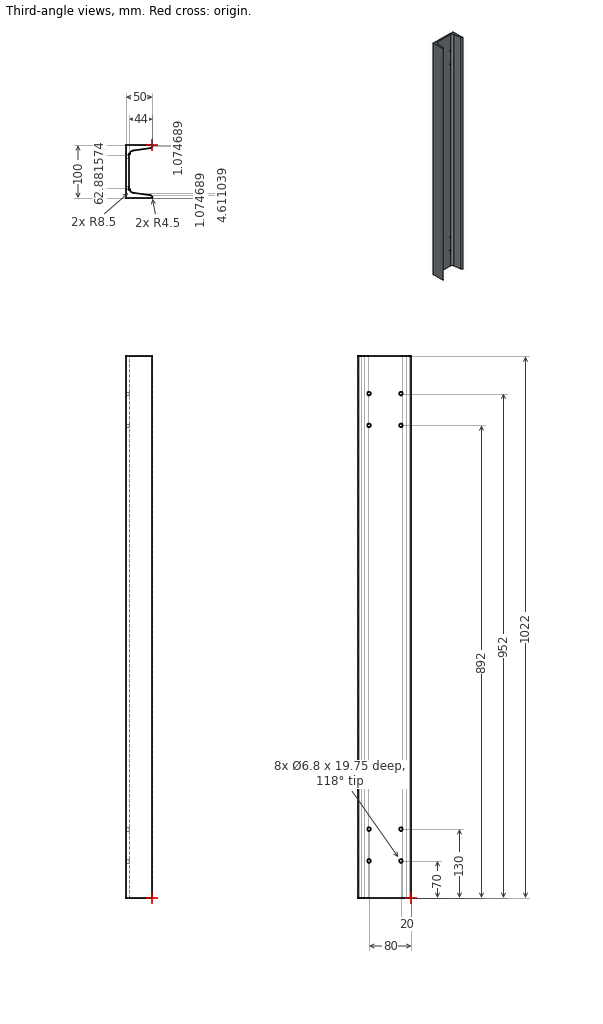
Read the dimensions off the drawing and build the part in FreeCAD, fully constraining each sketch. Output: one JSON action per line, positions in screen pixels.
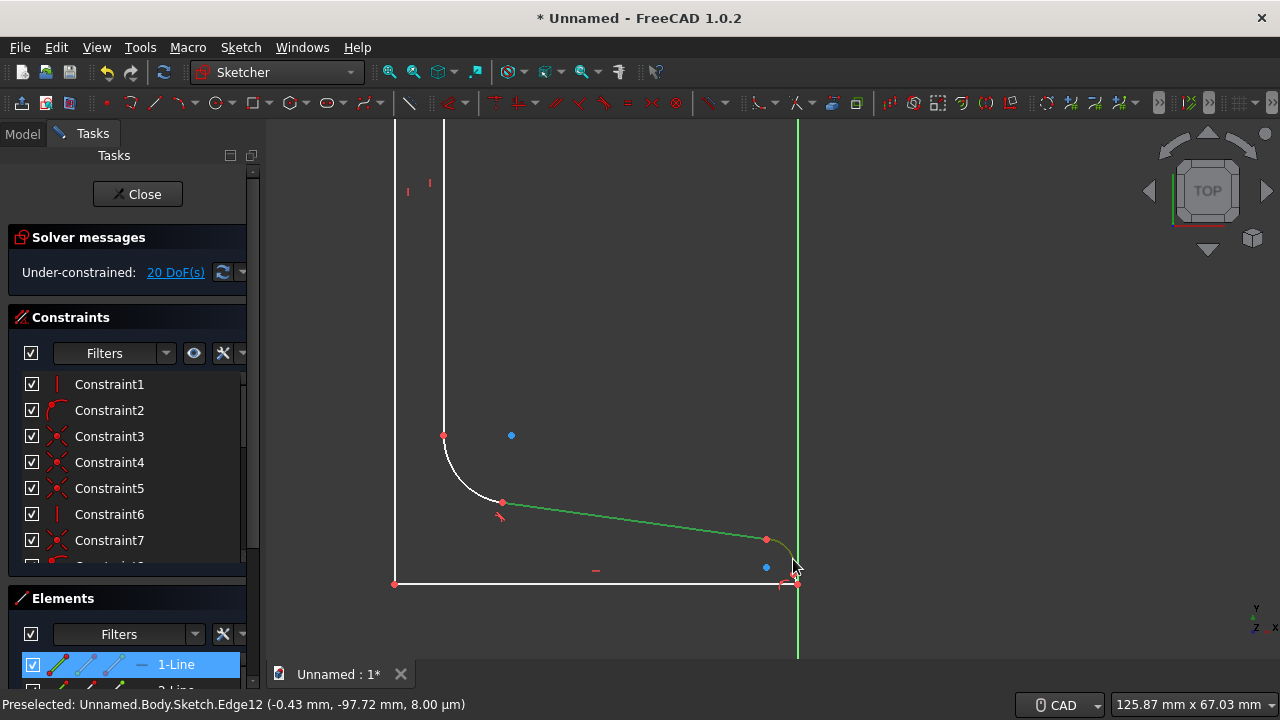
{"action": "key", "text": "t"}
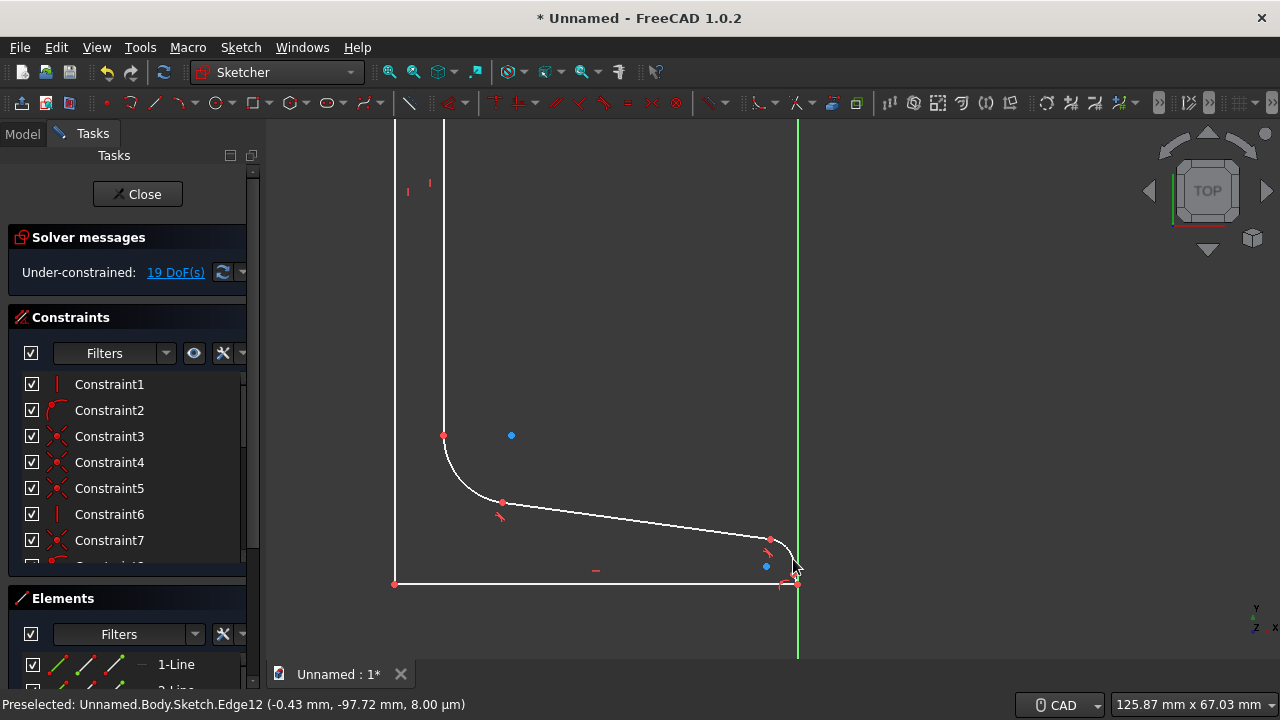
{"action": "left_click", "coordinate": [444, 283]}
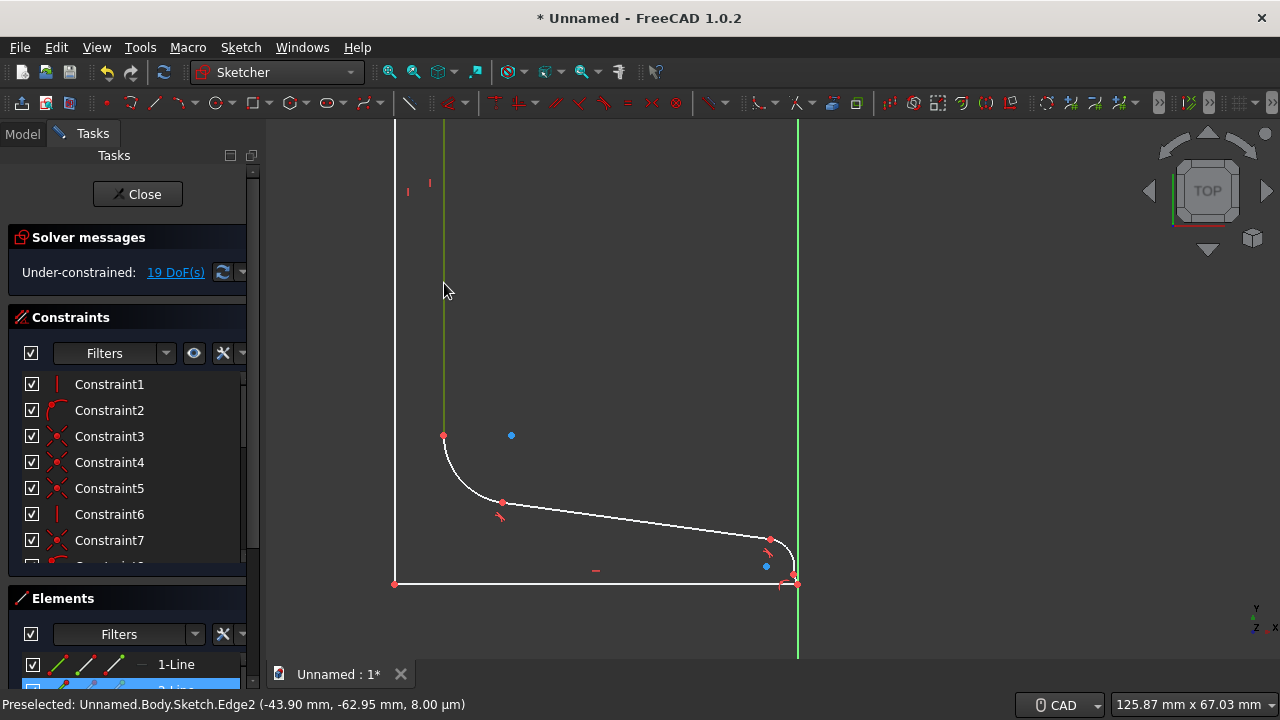
{"action": "left_click", "coordinate": [450, 464]}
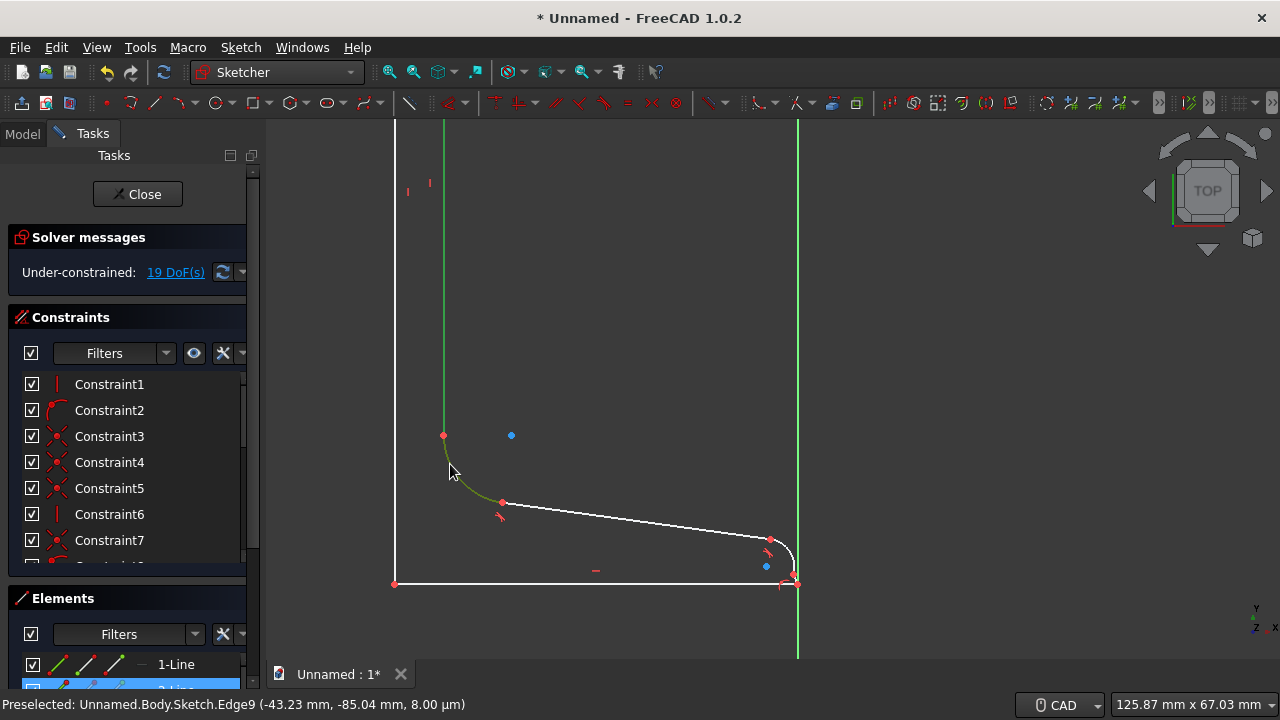
{"action": "left_click", "coordinate": [604, 104]}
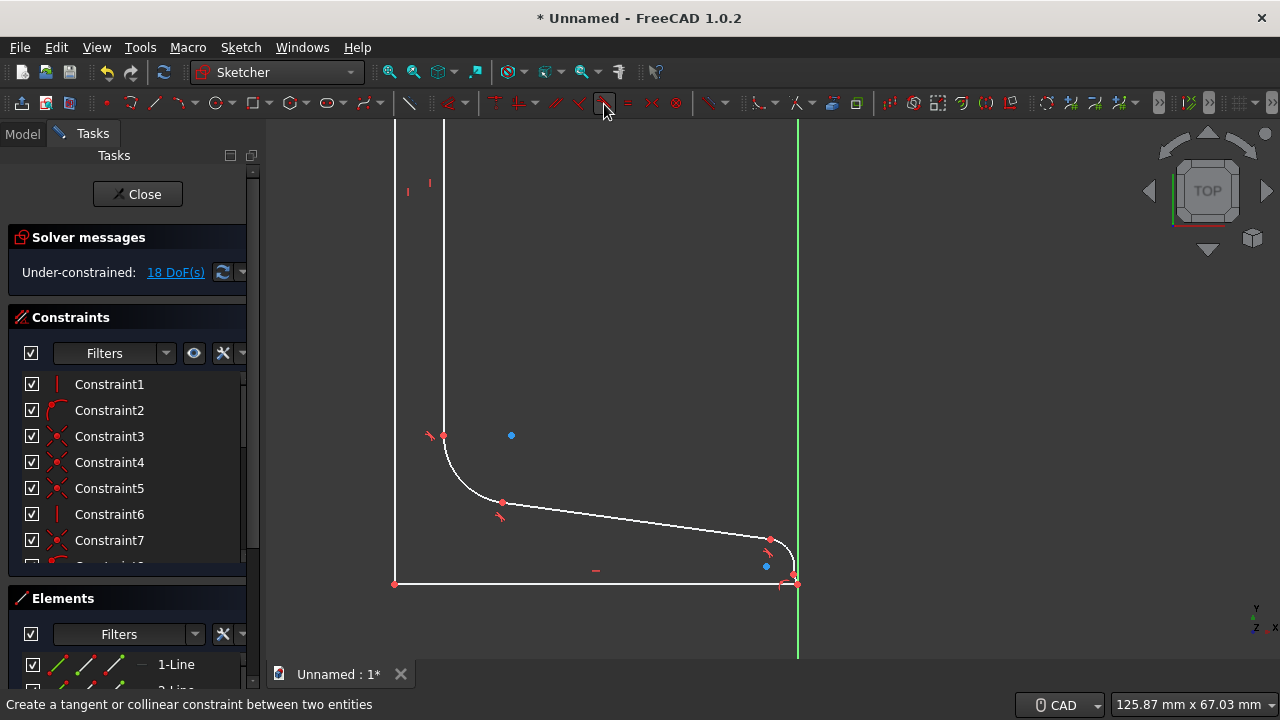
{"action": "left_click", "coordinate": [444, 283]}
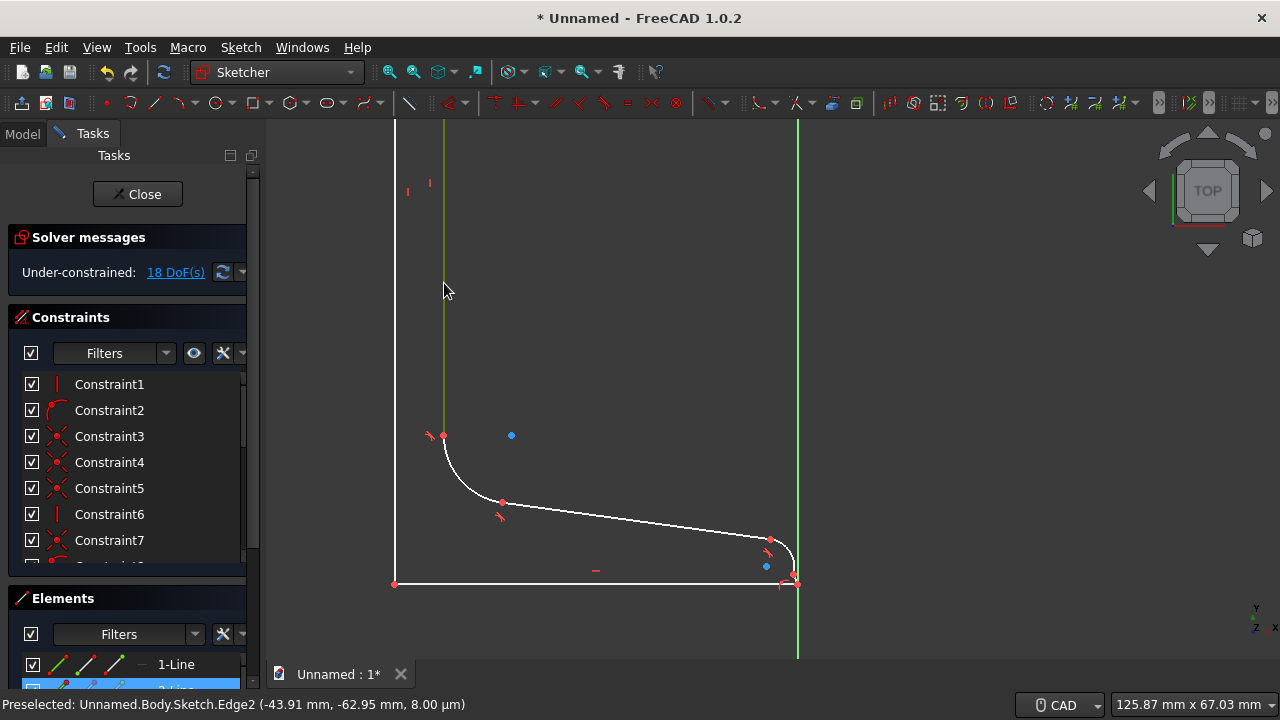
{"action": "scroll", "coordinate": [793, 560], "scroll_direction": "down", "scroll_amount": 4}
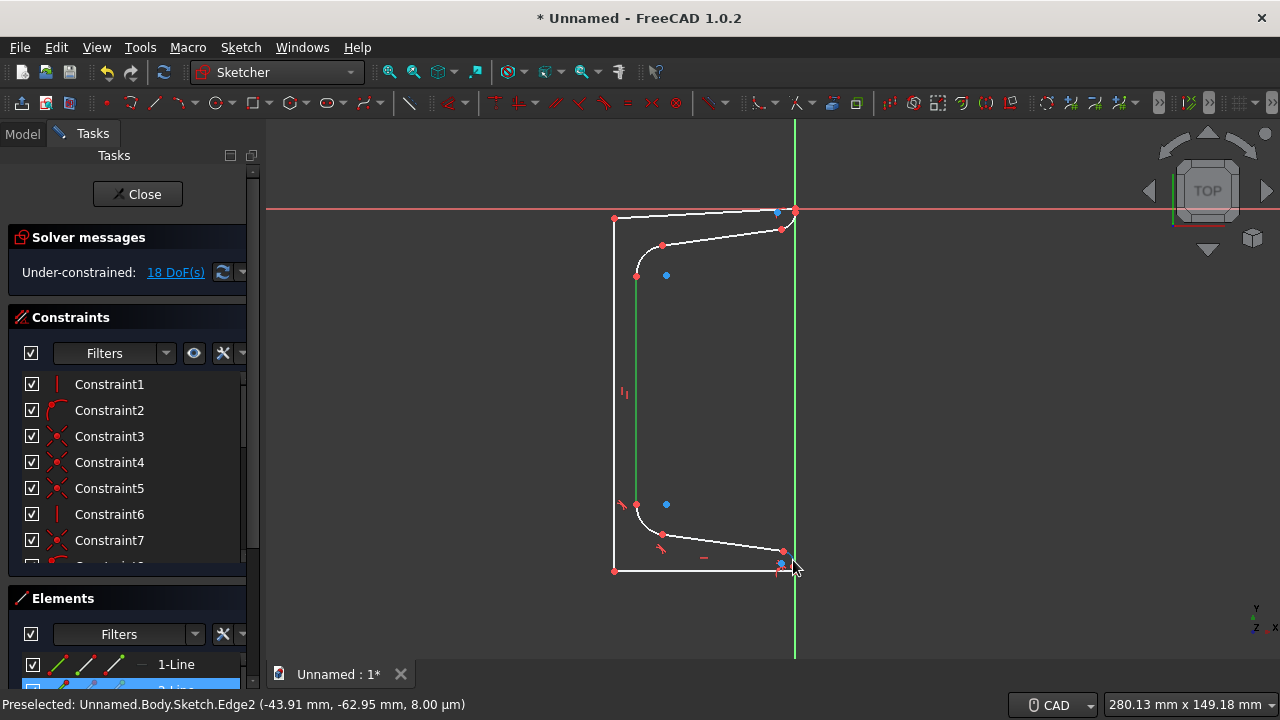
{"action": "left_click", "coordinate": [650, 250]}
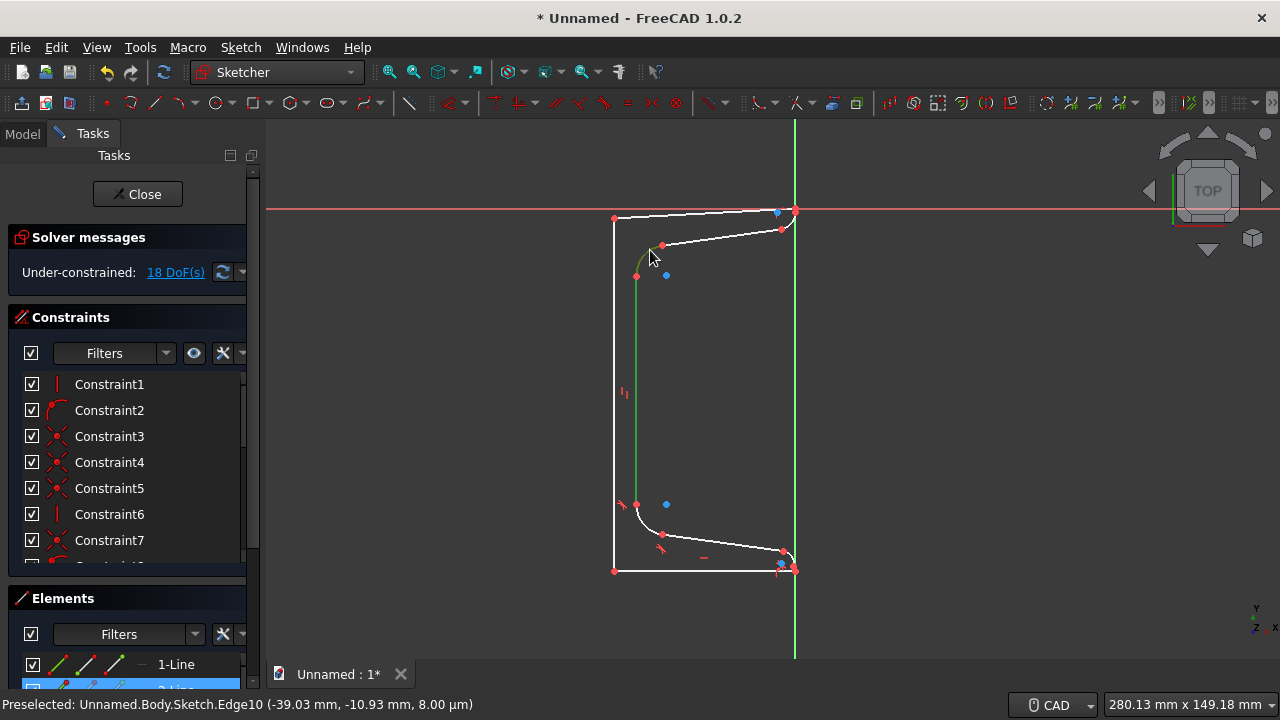
{"action": "left_click", "coordinate": [604, 104]}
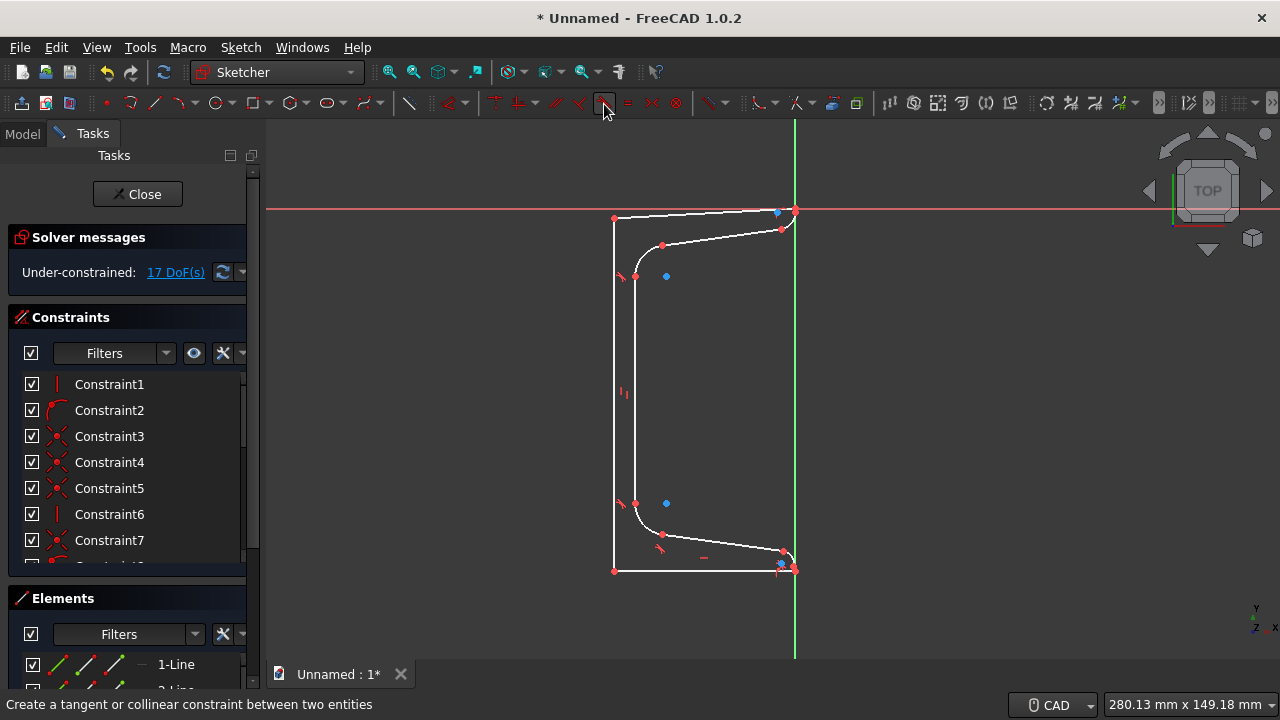
{"action": "left_click", "coordinate": [698, 241]}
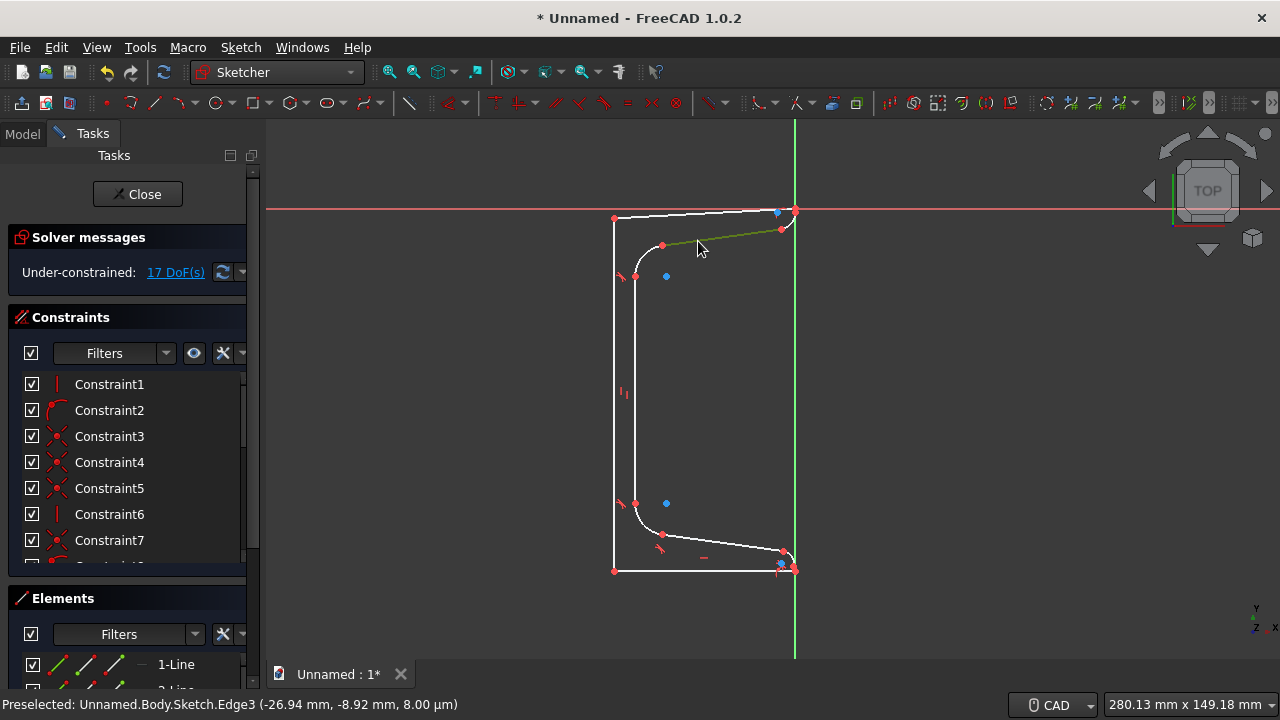
{"action": "left_click", "coordinate": [650, 250]}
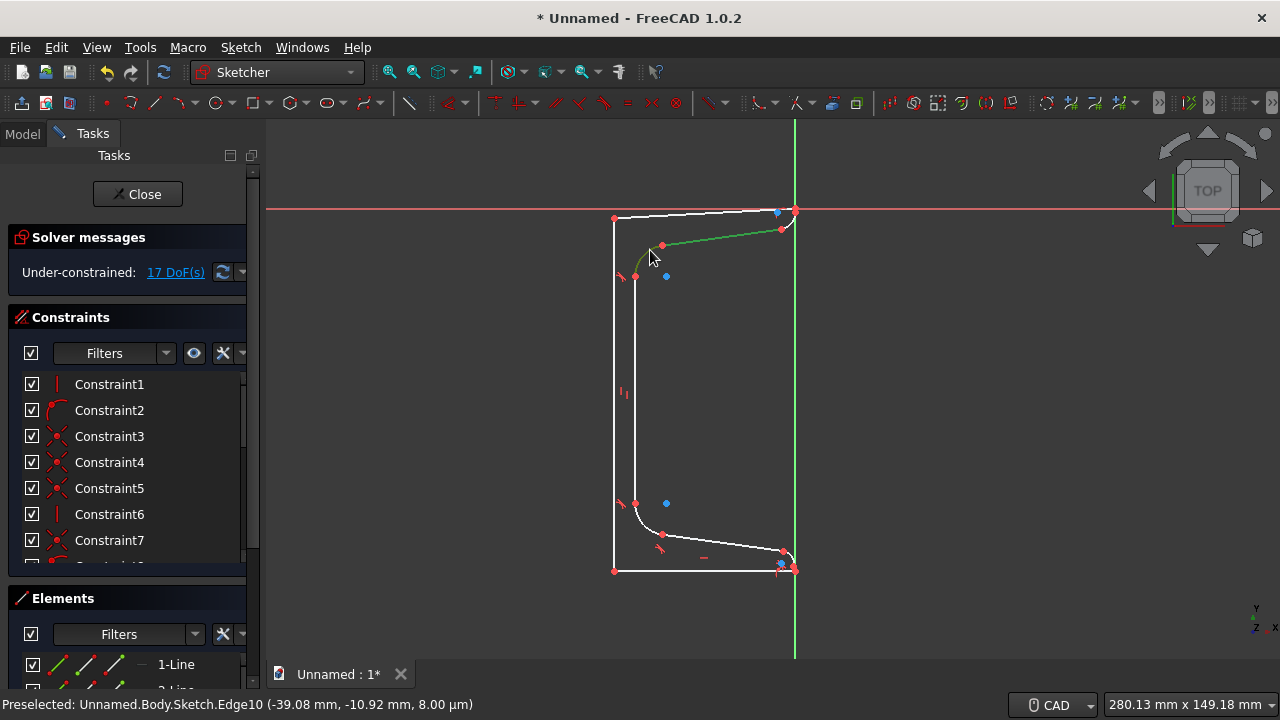
{"action": "left_click", "coordinate": [604, 104]}